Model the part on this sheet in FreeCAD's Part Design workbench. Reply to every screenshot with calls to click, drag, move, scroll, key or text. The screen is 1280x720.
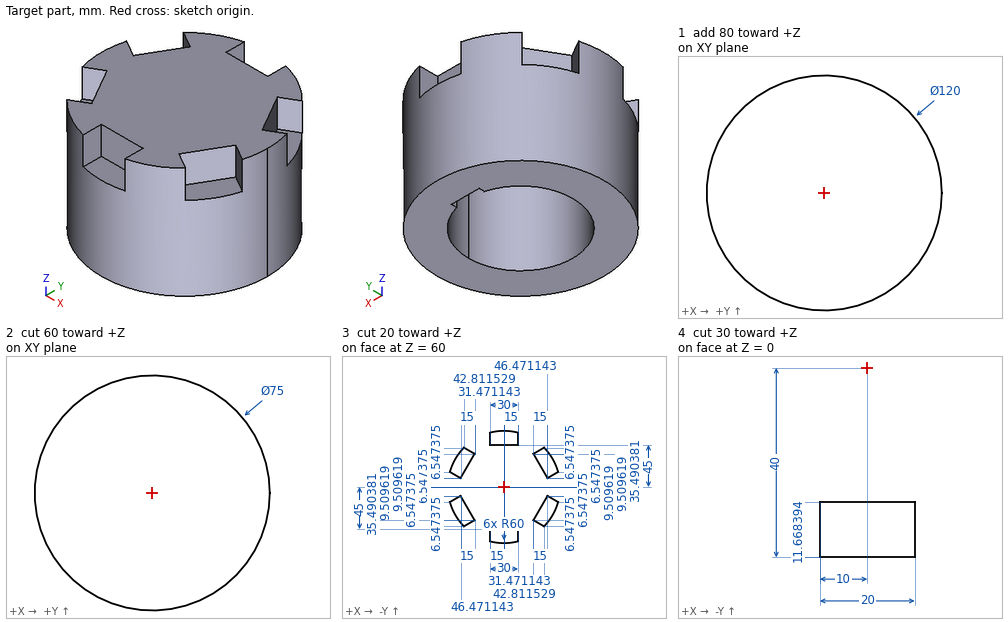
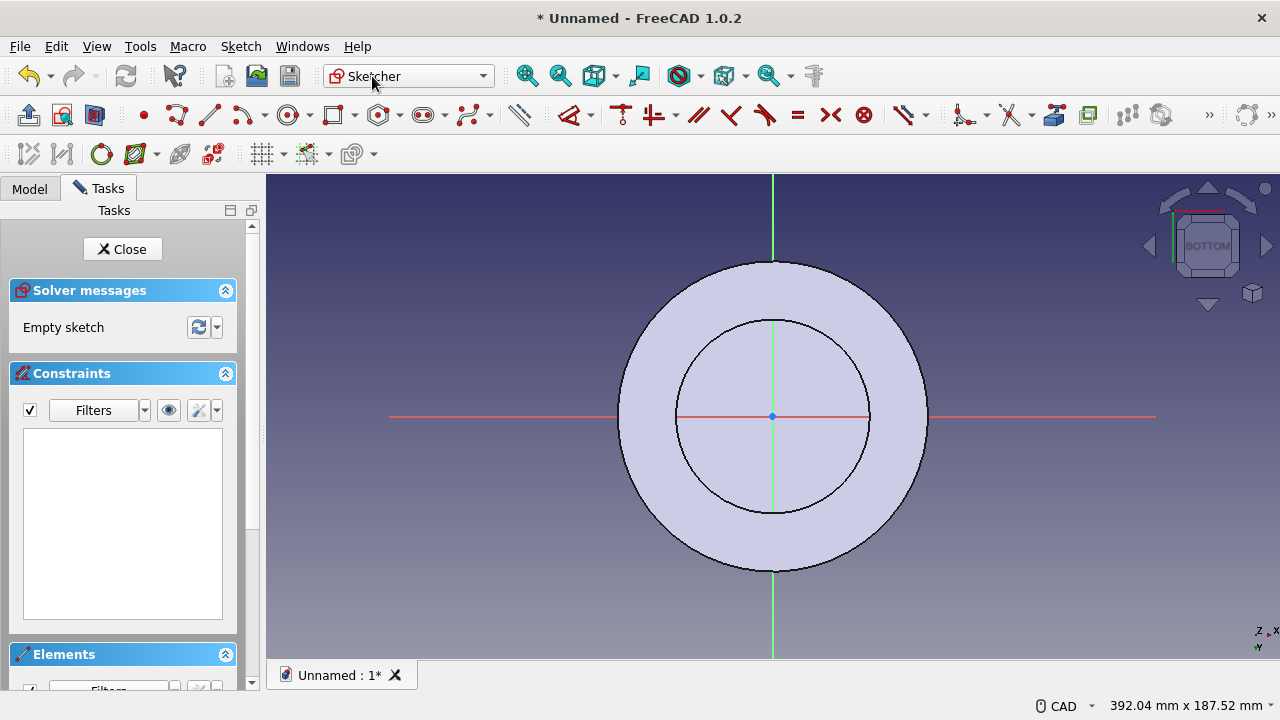
click(177, 116)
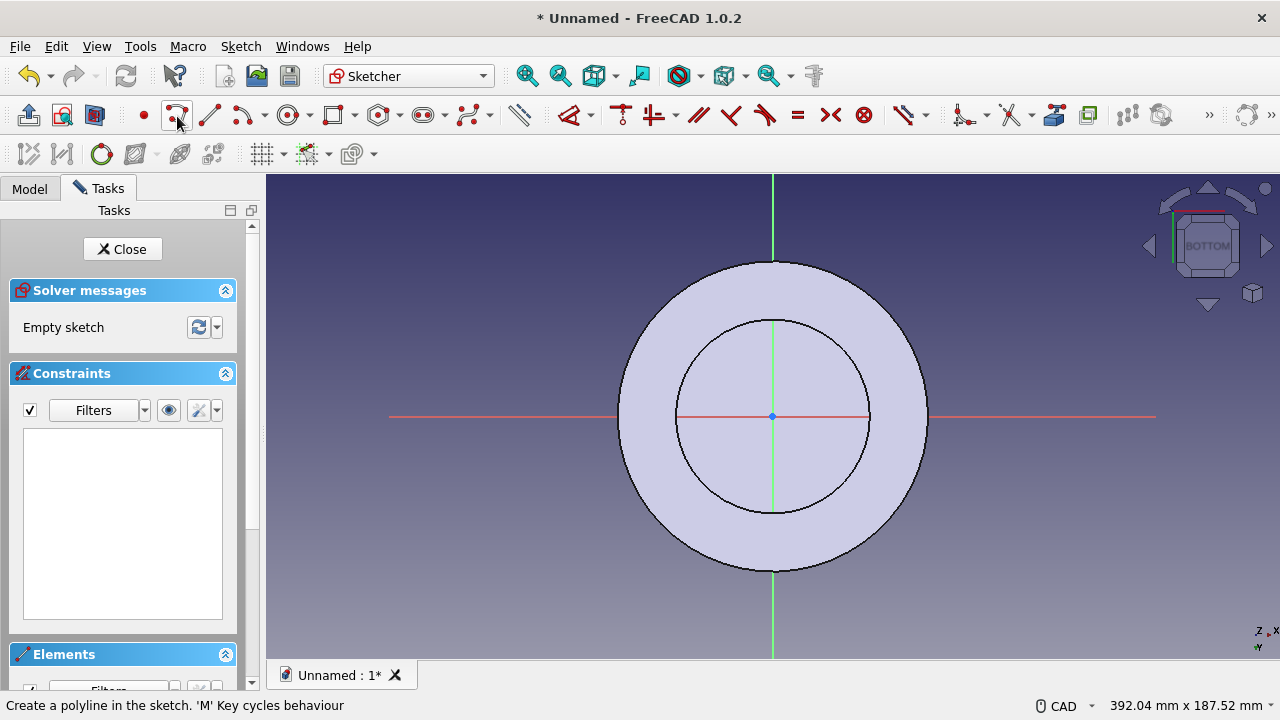
click(884, 525)
click(854, 508)
click(893, 441)
click(922, 458)
right_click(922, 458)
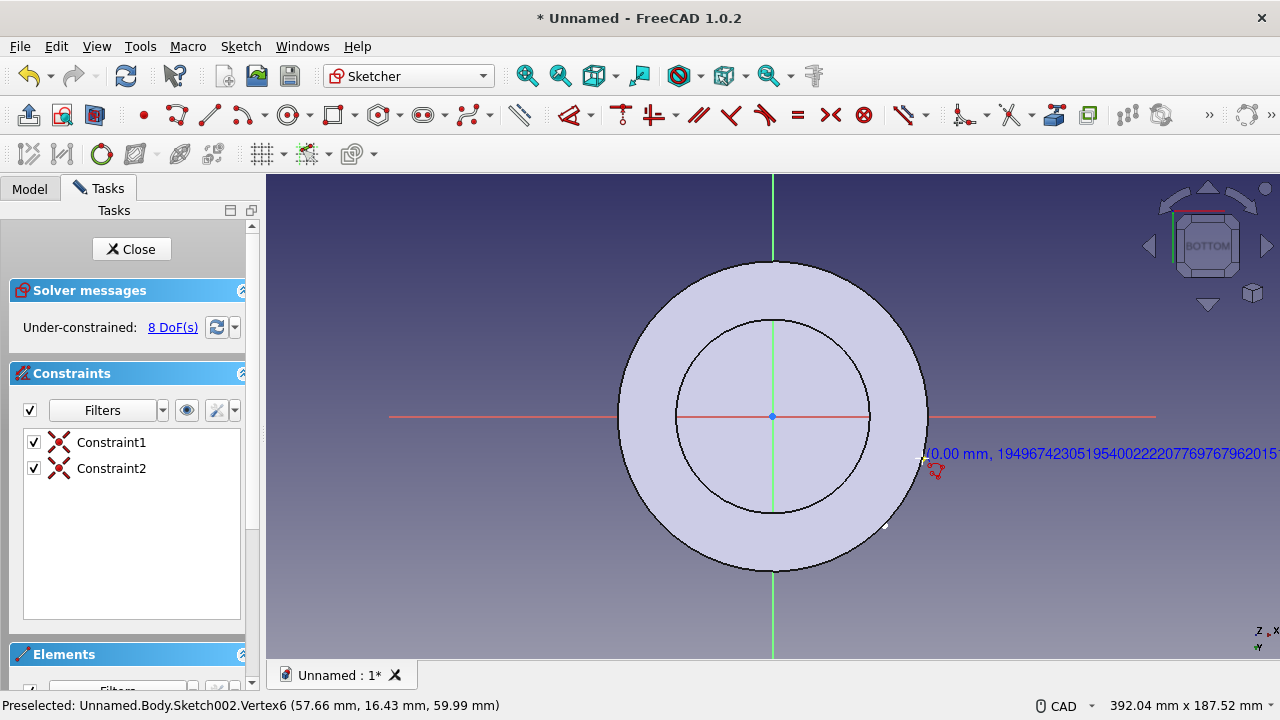
key(g)
key(3)
key(a)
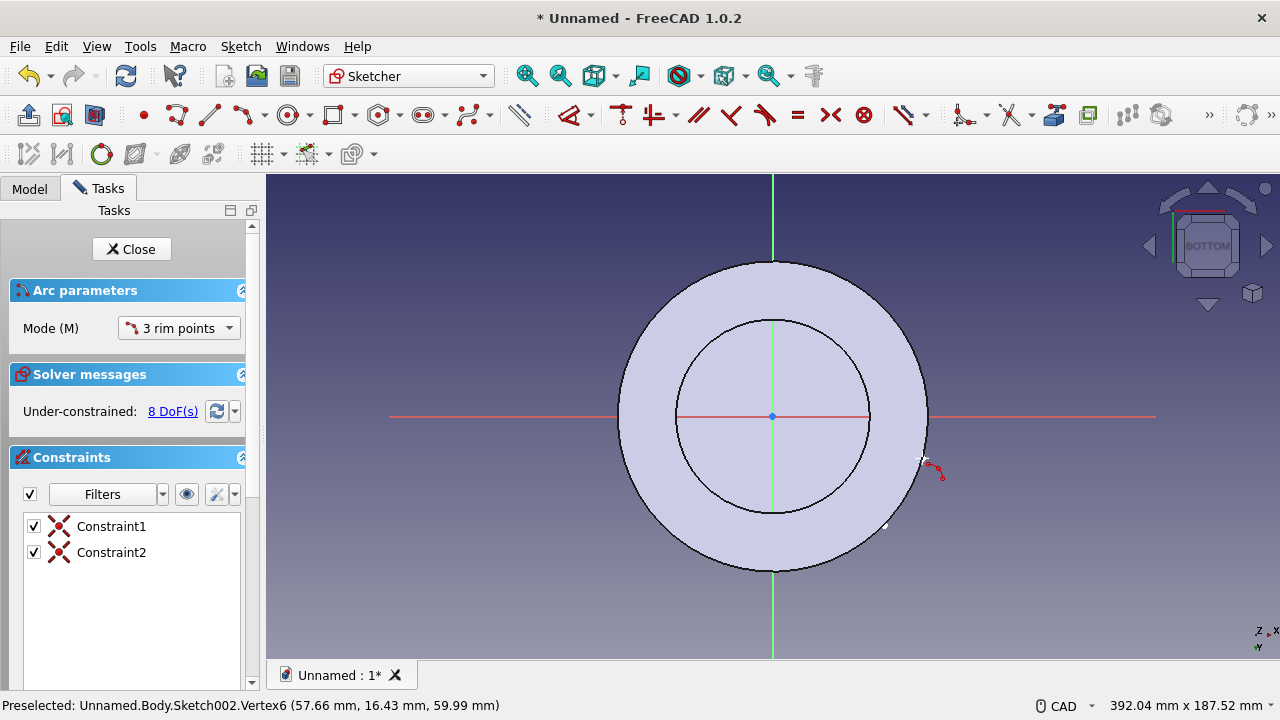
click(922, 459)
click(884, 526)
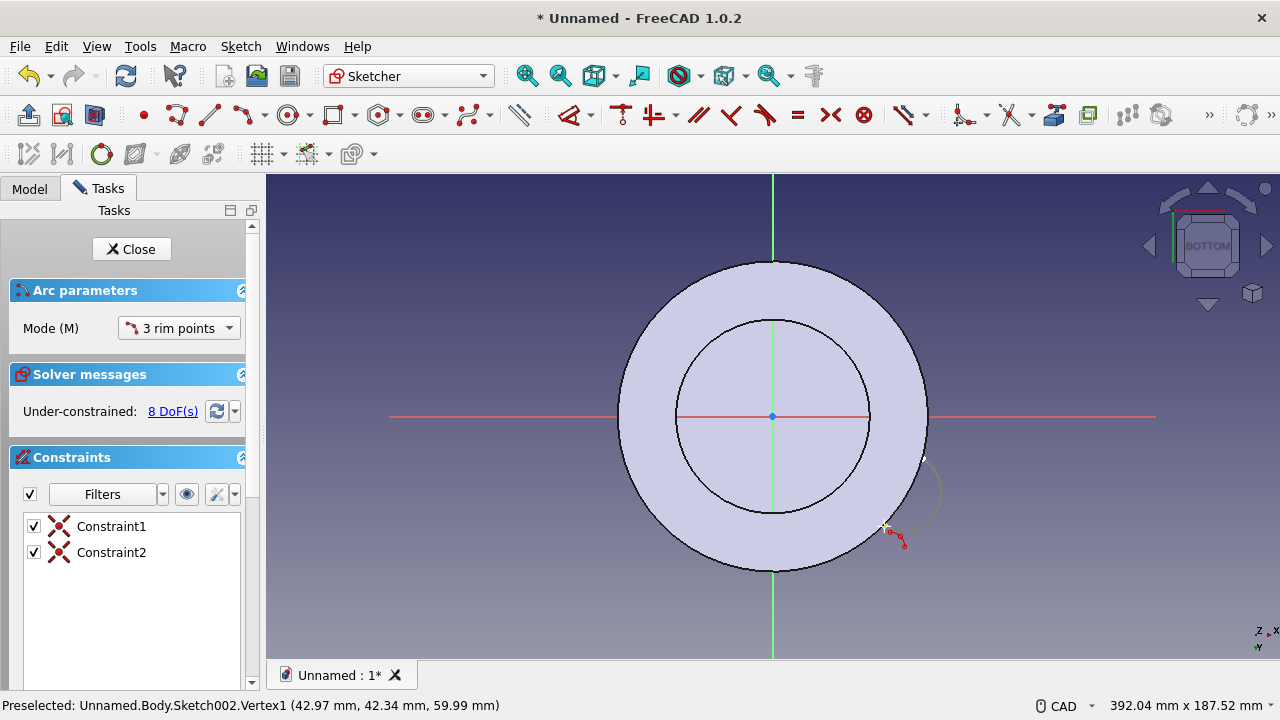
scroll(907, 494, up, 6)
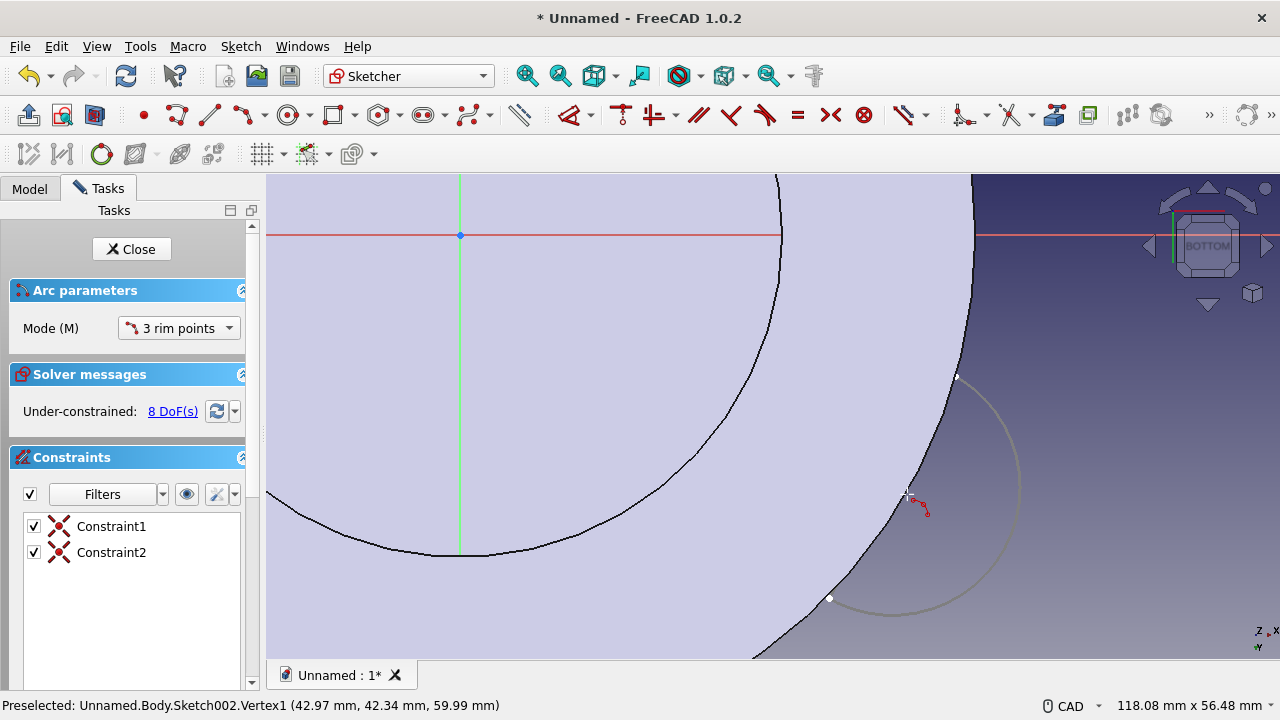
click(906, 493)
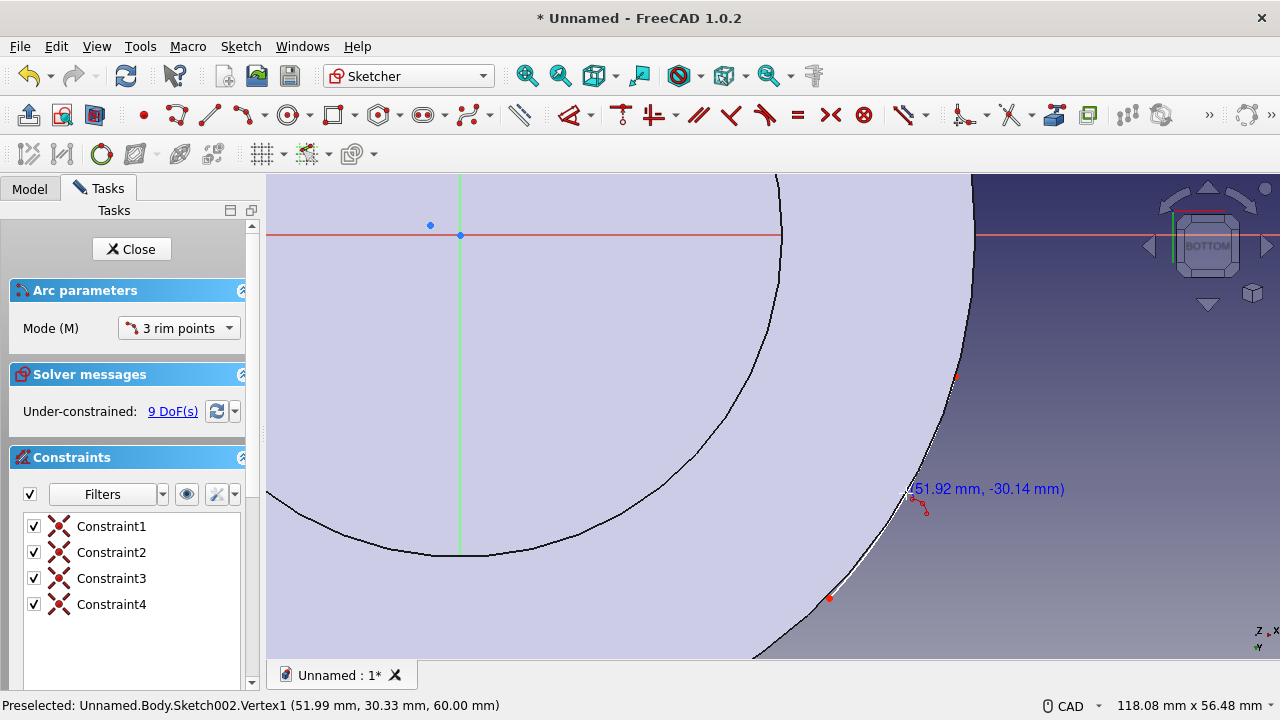
click(177, 116)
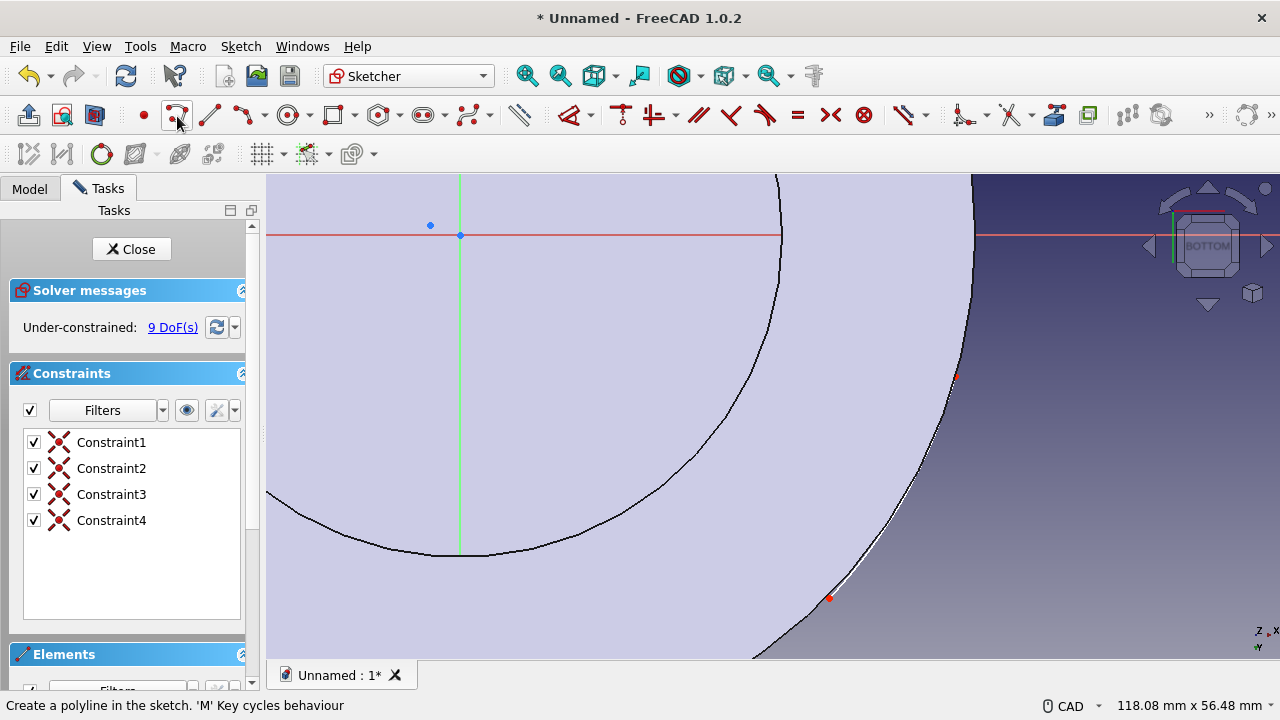
scroll(810, 495, down, 6)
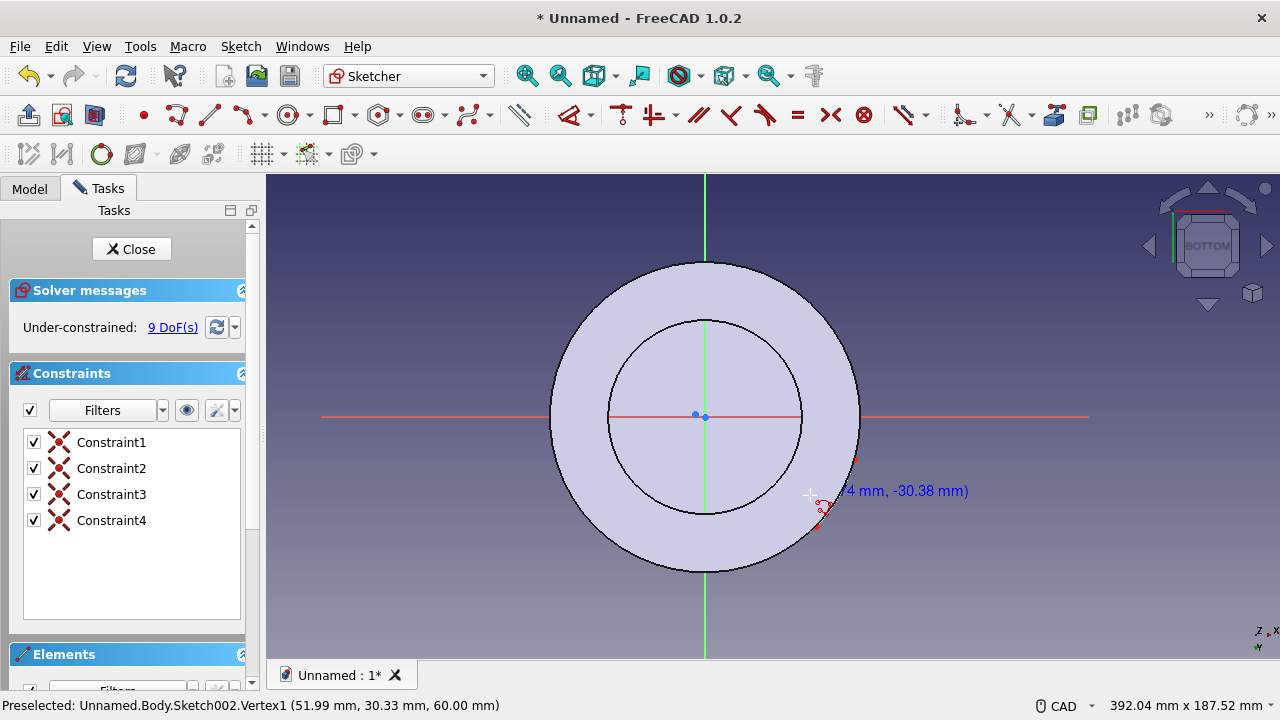
click(666, 567)
click(666, 534)
click(744, 534)
click(744, 567)
right_click(744, 567)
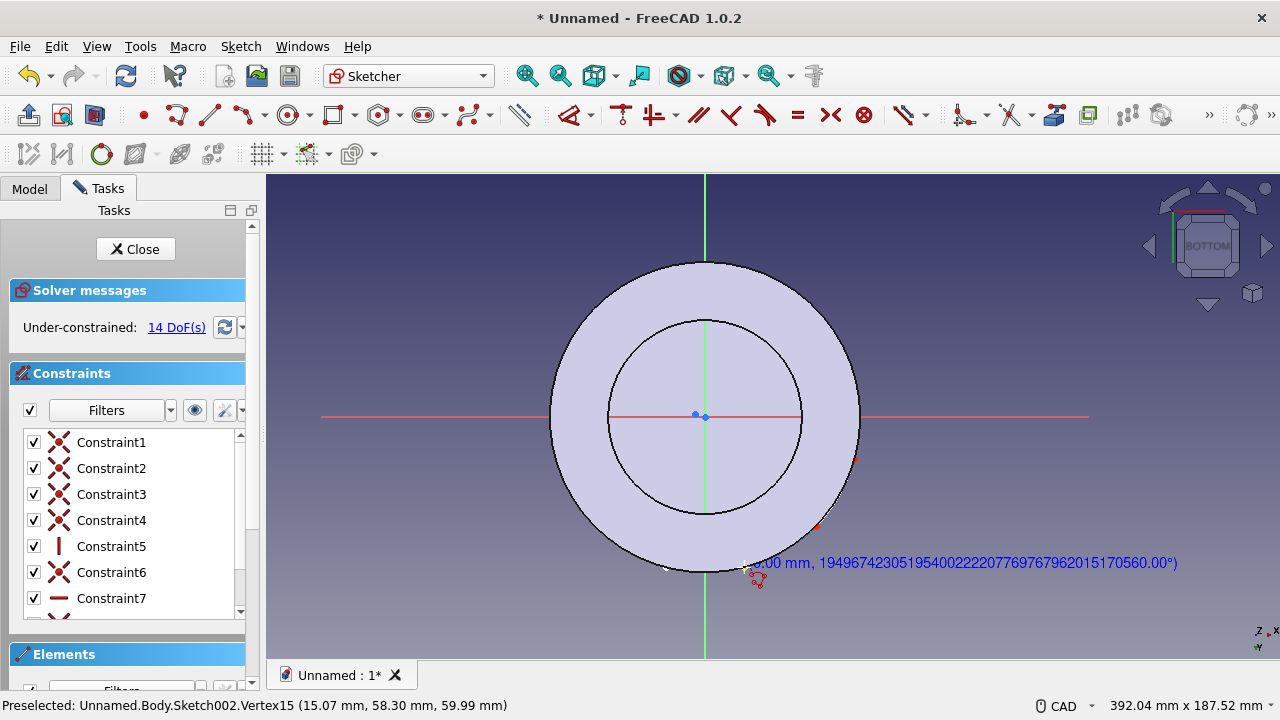
click(242, 116)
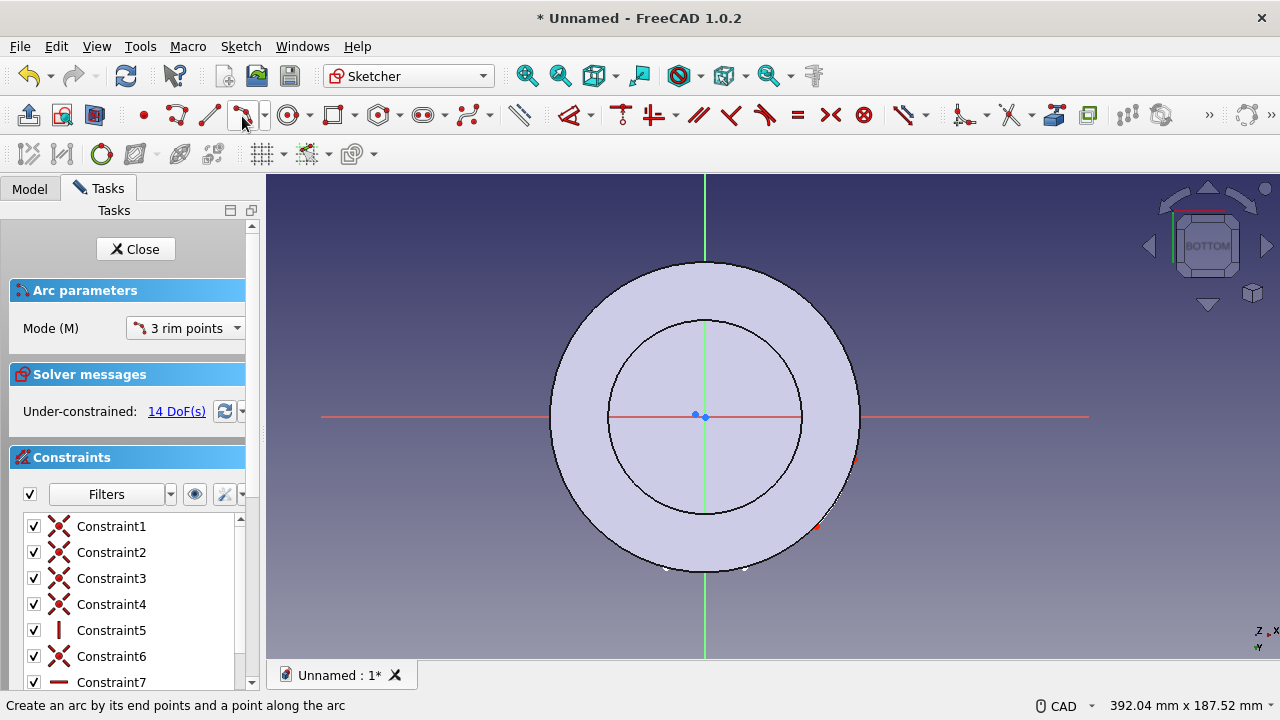
click(744, 568)
click(666, 568)